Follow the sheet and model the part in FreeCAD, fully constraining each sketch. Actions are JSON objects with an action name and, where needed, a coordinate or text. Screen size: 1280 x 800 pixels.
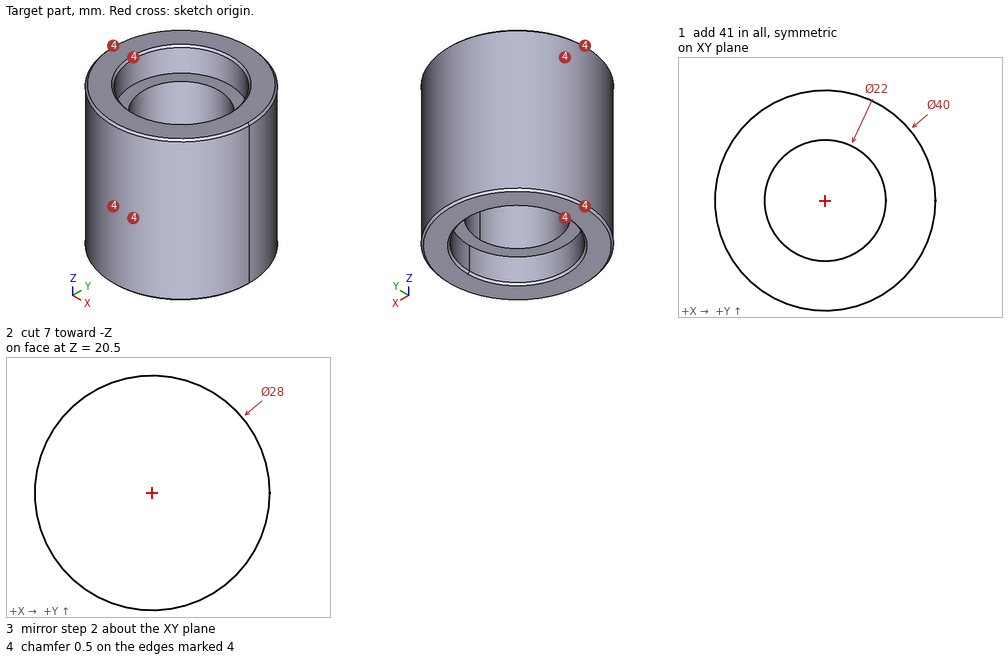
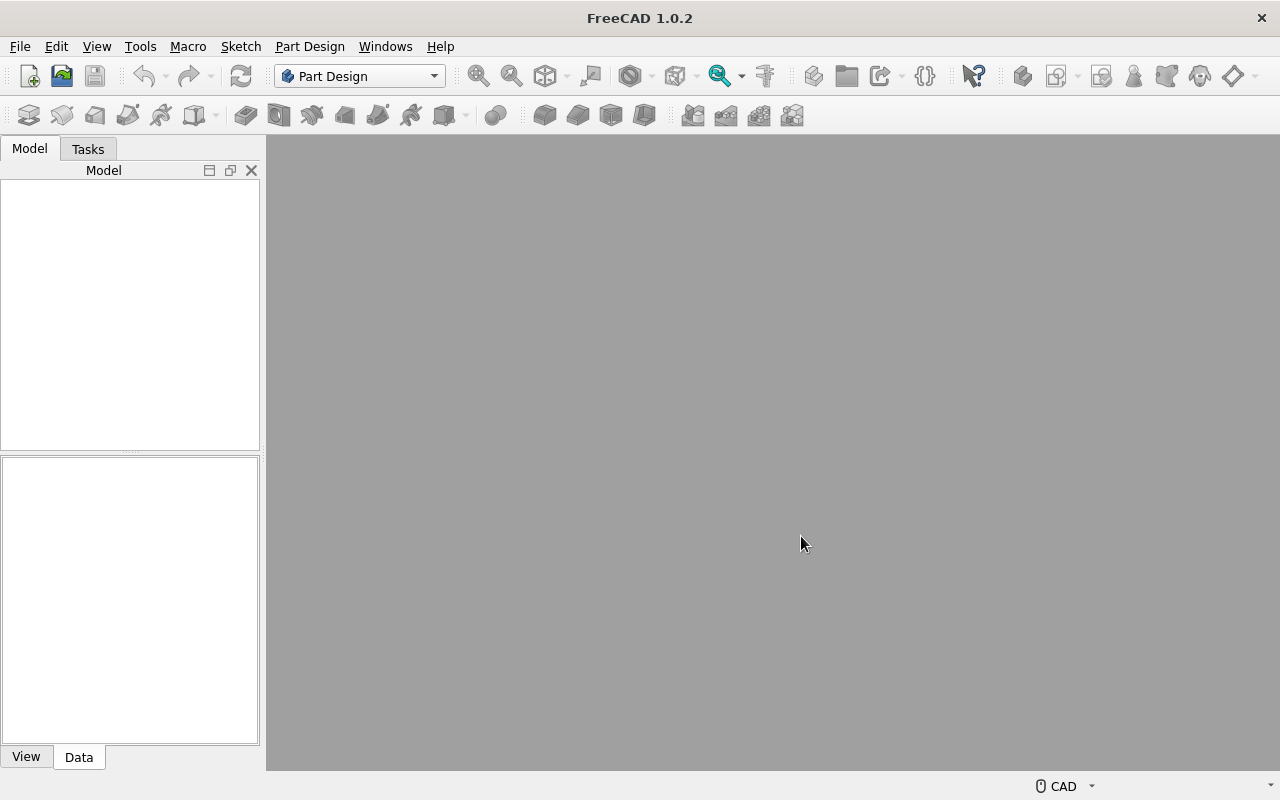
{"action": "left_click", "coordinate": [29, 76]}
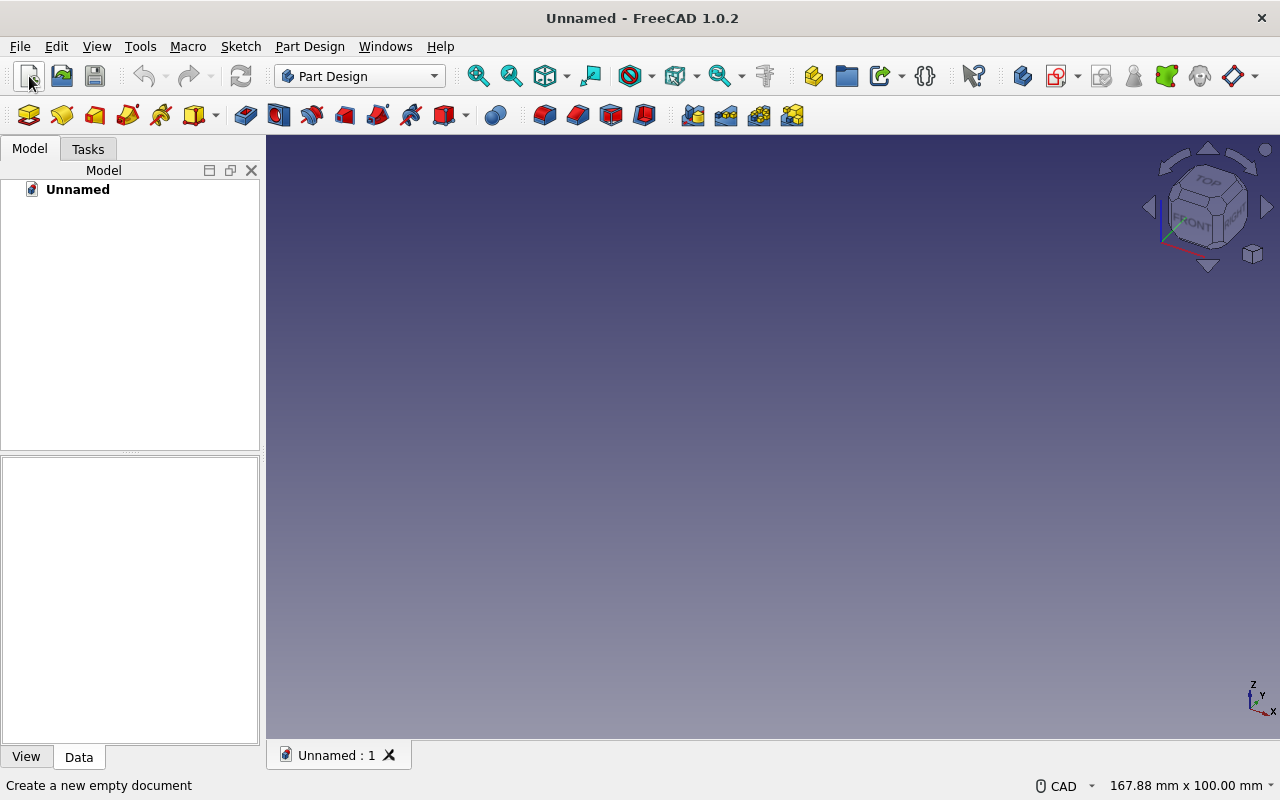
{"action": "left_click", "coordinate": [1056, 76]}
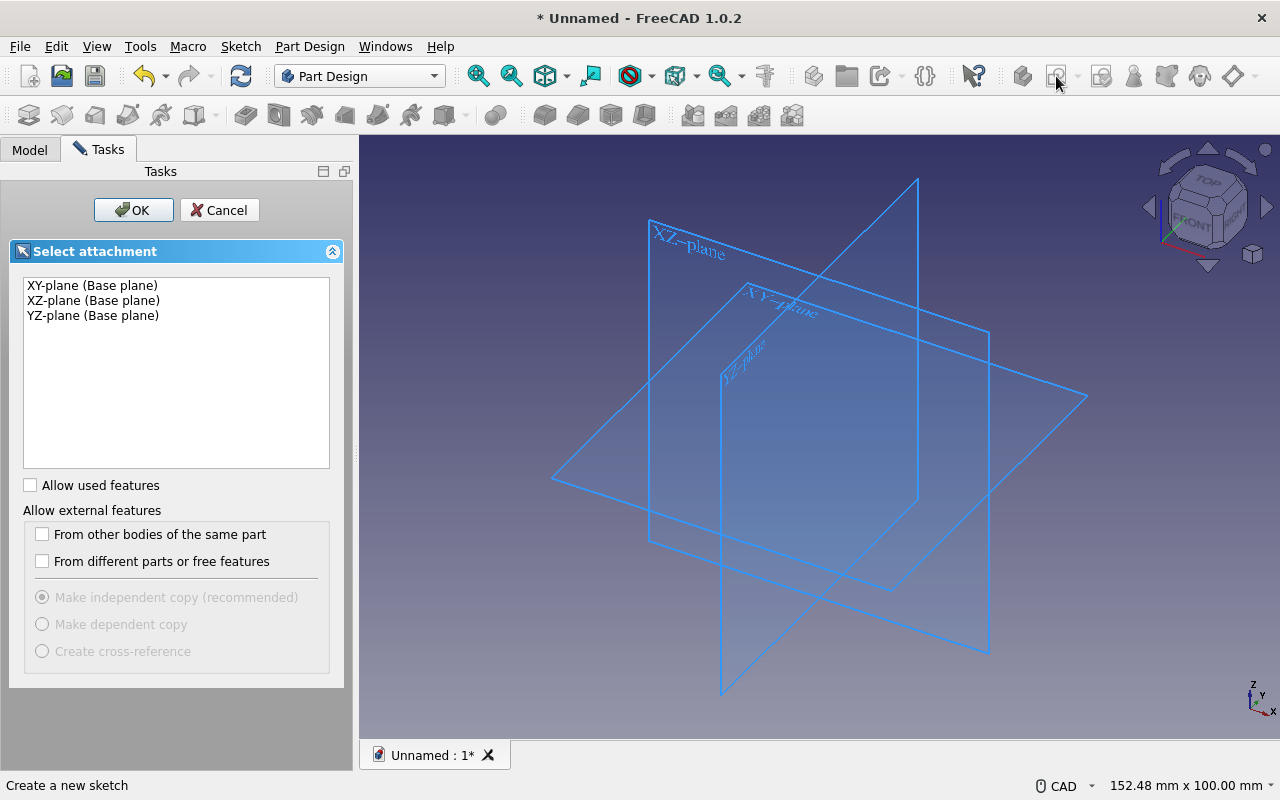
{"action": "left_click", "coordinate": [84, 286]}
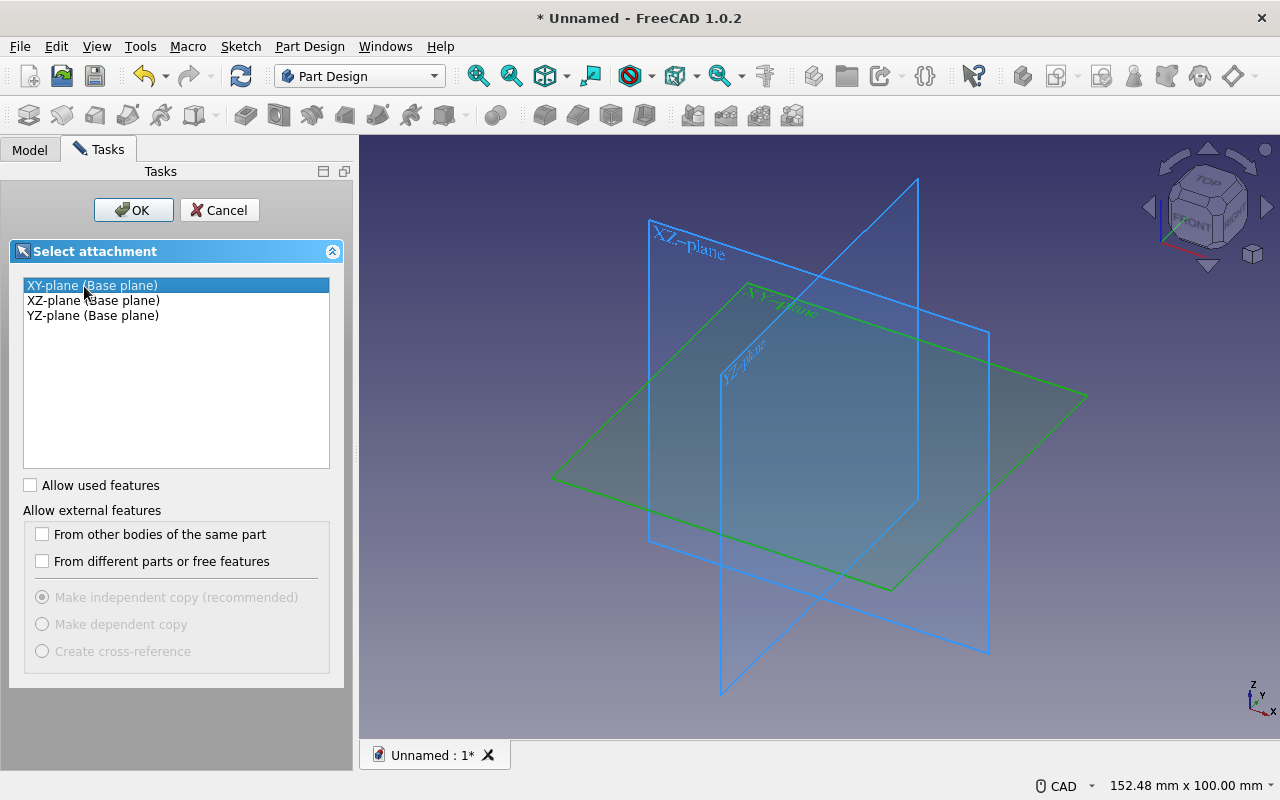
{"action": "left_click", "coordinate": [134, 210]}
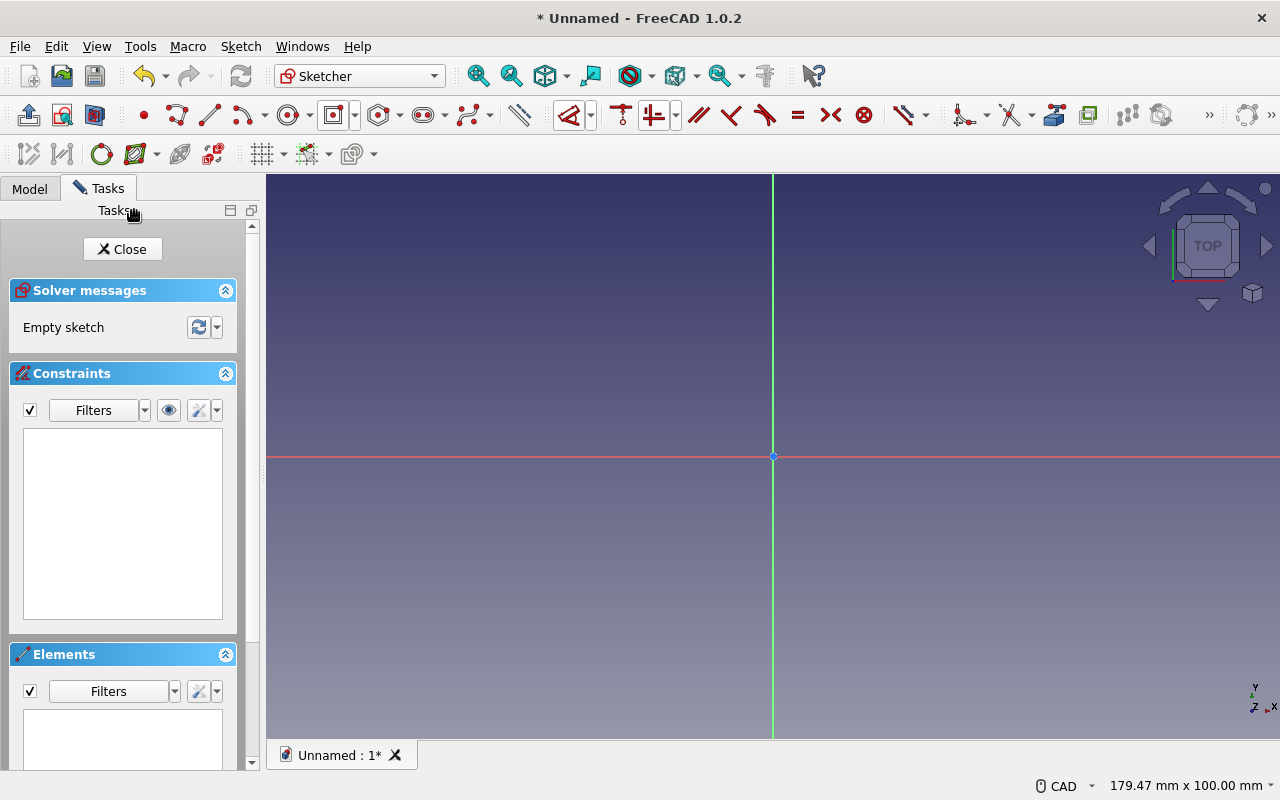
{"action": "scroll", "coordinate": [912, 456], "scroll_direction": "up", "scroll_amount": 2}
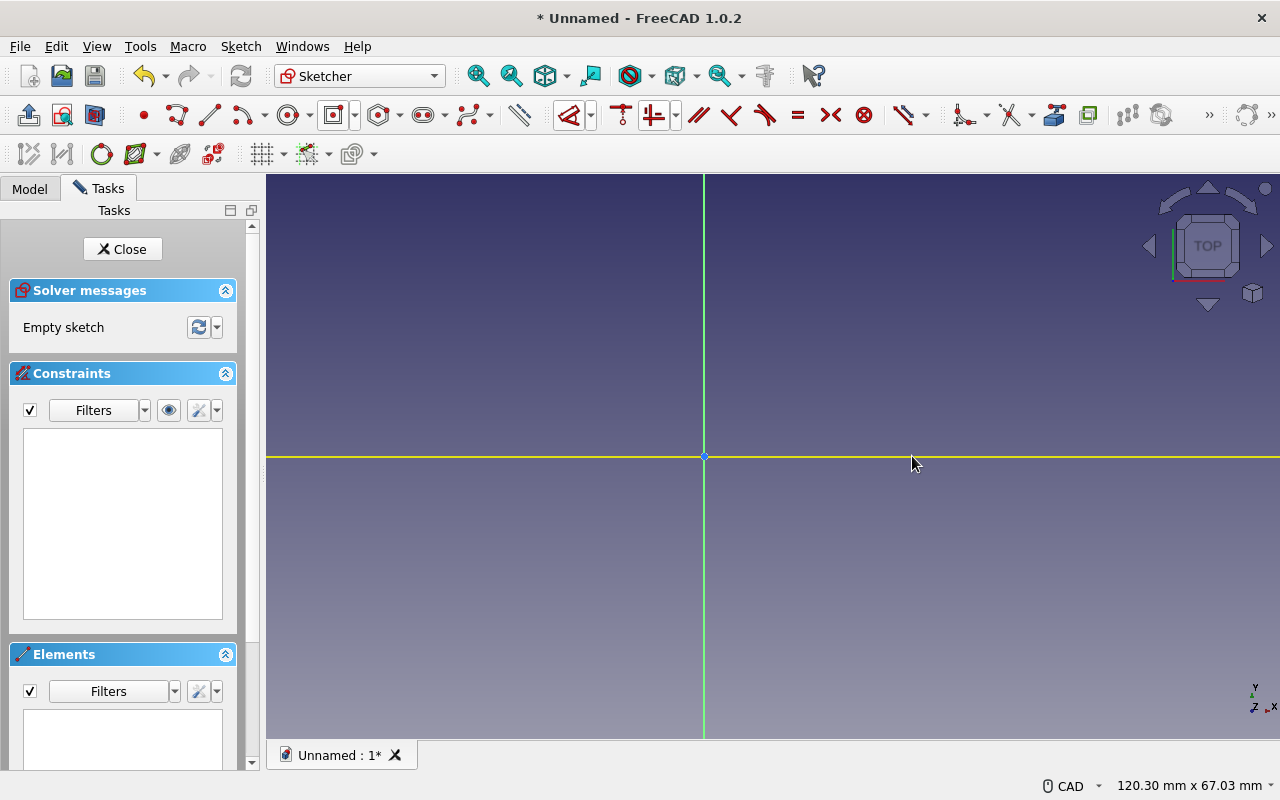
{"action": "left_click", "coordinate": [288, 116]}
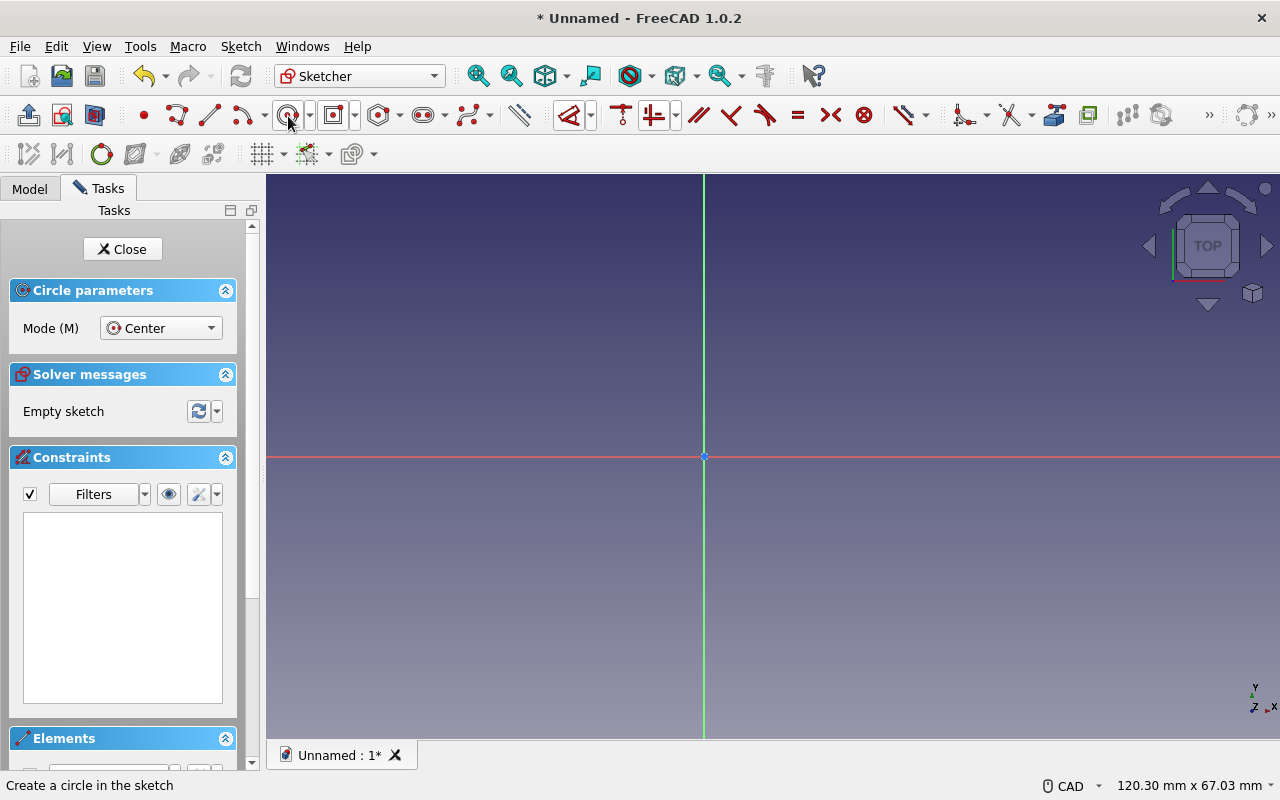
{"action": "left_click", "coordinate": [704, 456]}
{"action": "mouse_move", "coordinate": [824, 337]}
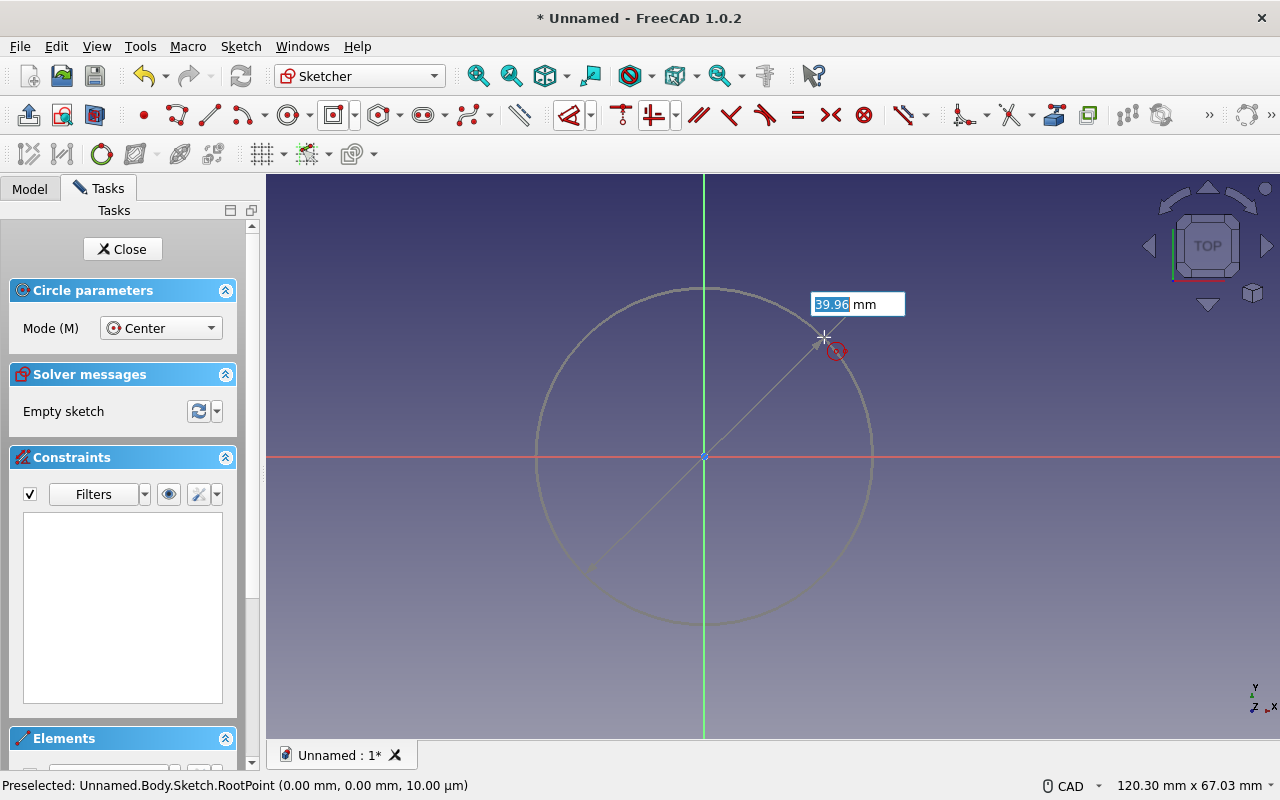
{"action": "type", "text": "40"}
{"action": "key", "text": "Return"}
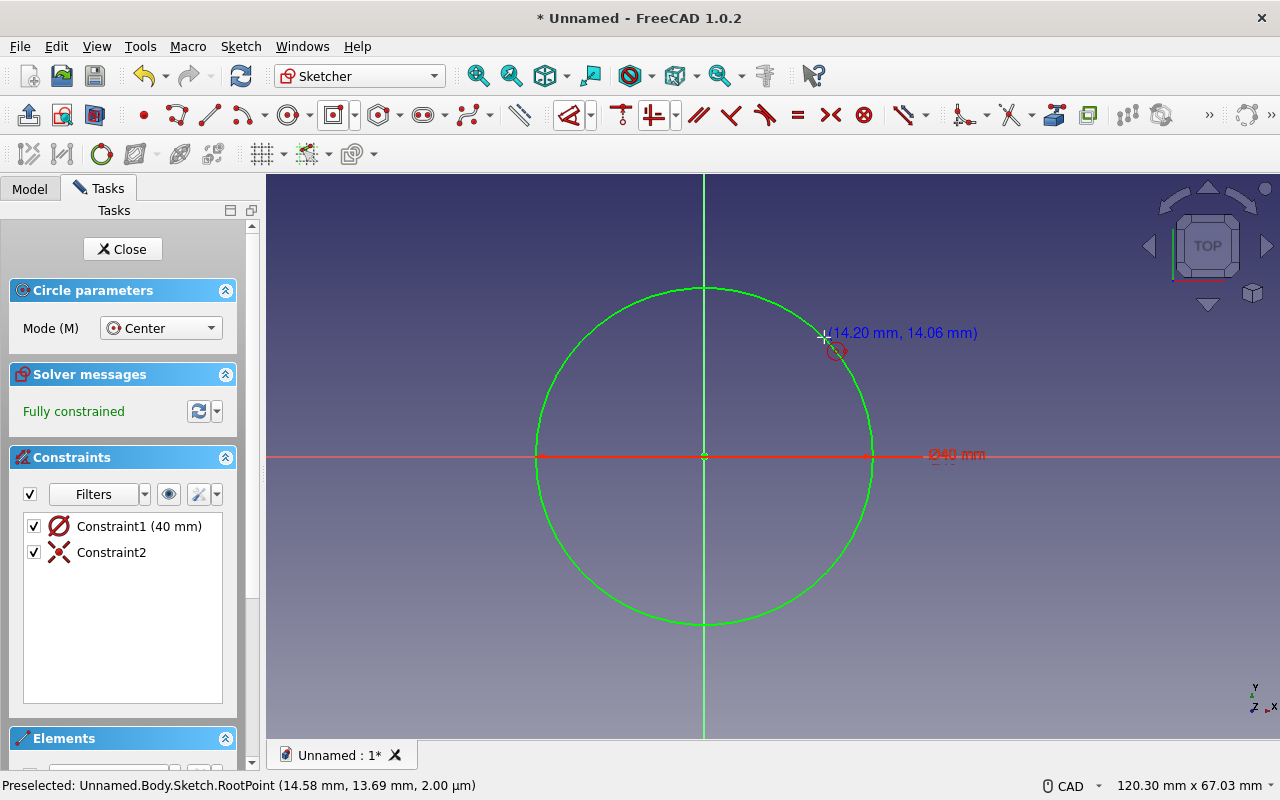
{"action": "left_click", "coordinate": [704, 456]}
{"action": "mouse_move", "coordinate": [770, 391]}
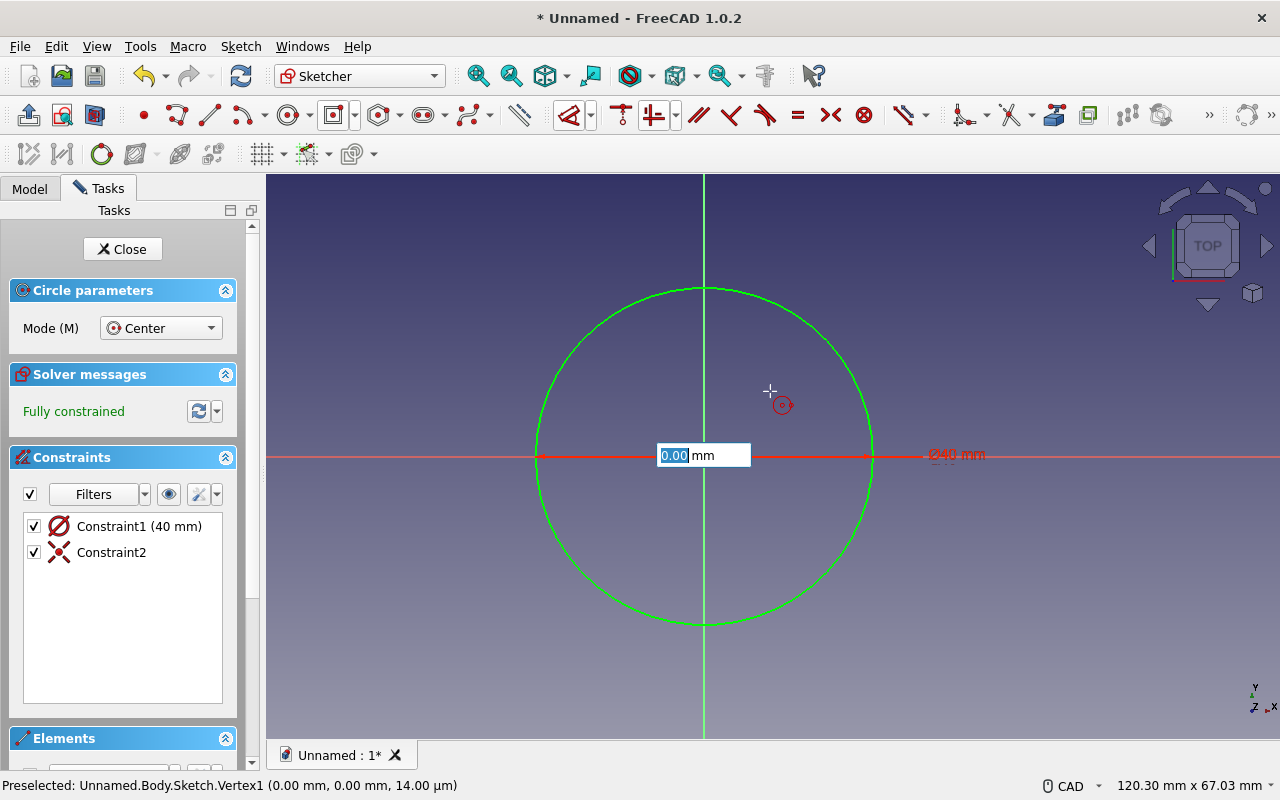
{"action": "type", "text": "22"}
{"action": "key", "text": "Return"}
{"action": "key", "text": "Escape"}